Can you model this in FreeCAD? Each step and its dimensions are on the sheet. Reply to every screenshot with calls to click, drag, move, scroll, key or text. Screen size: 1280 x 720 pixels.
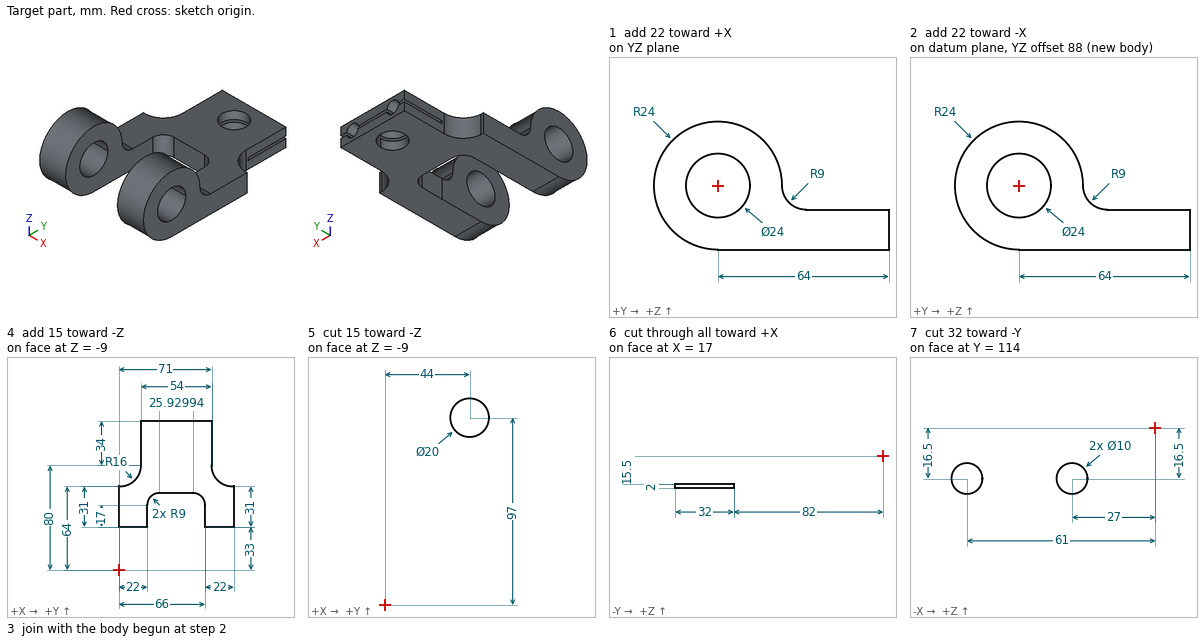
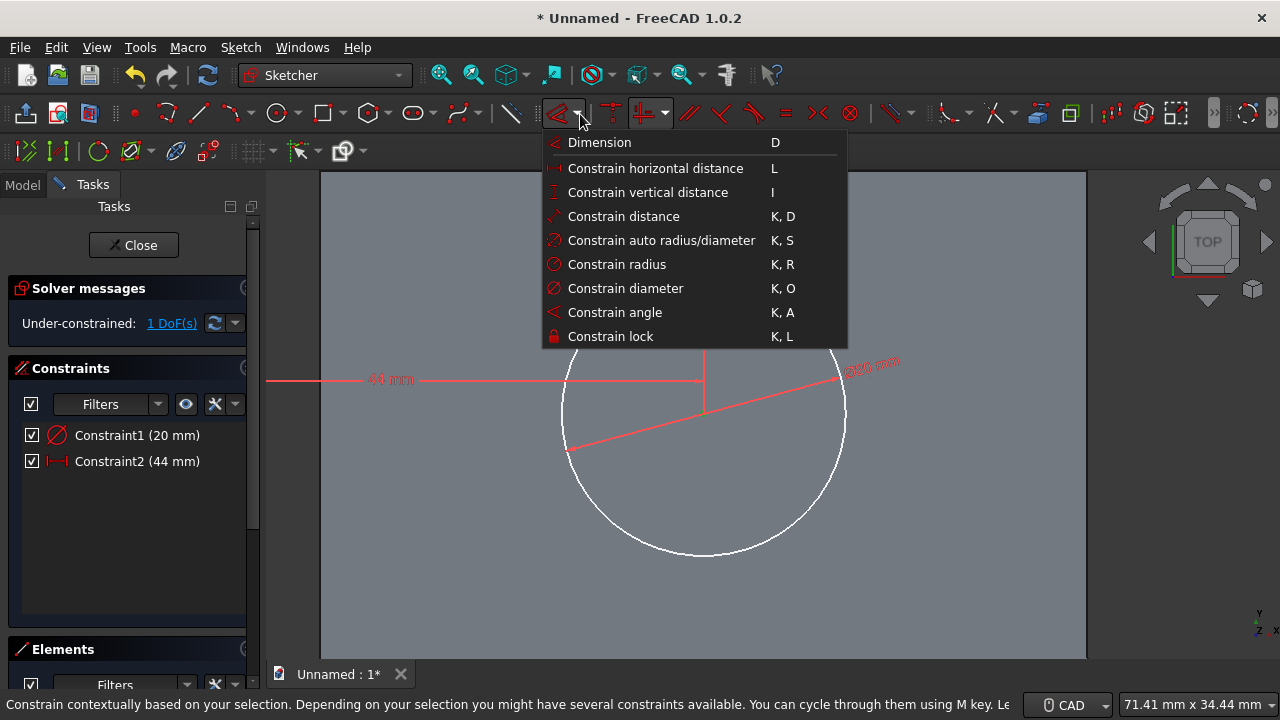
click(695, 192)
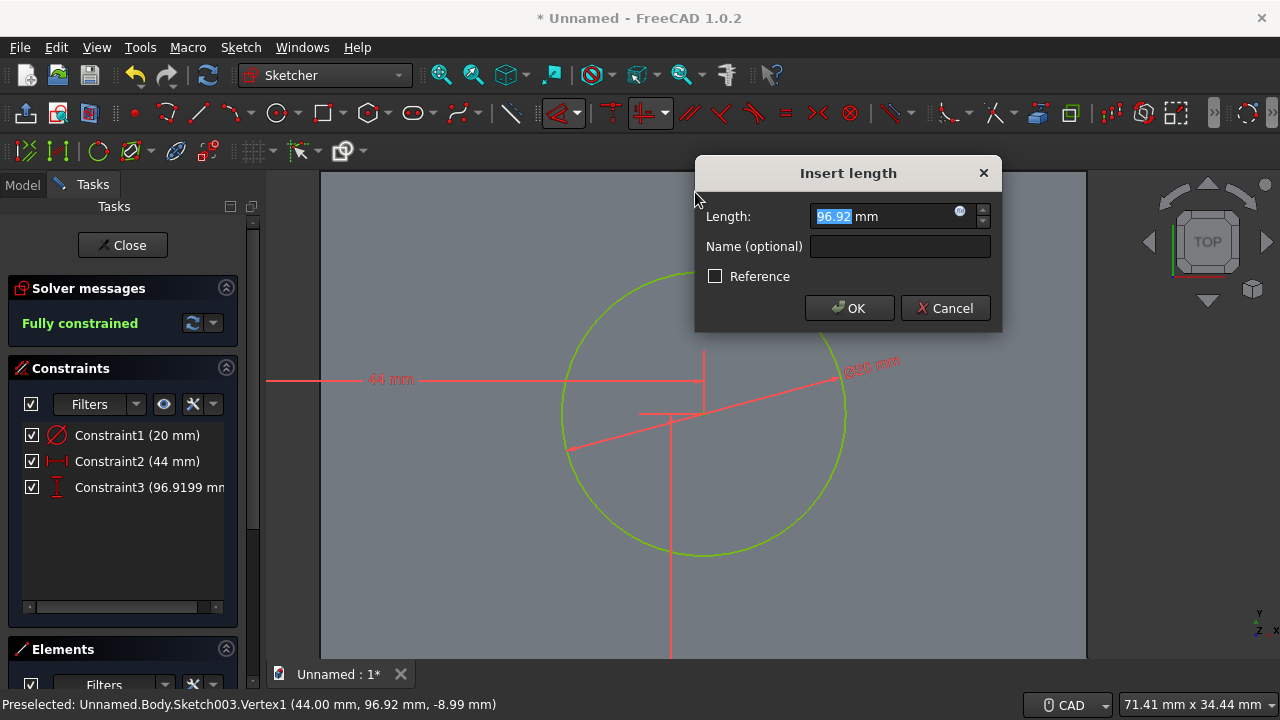
text(97)
key(Return)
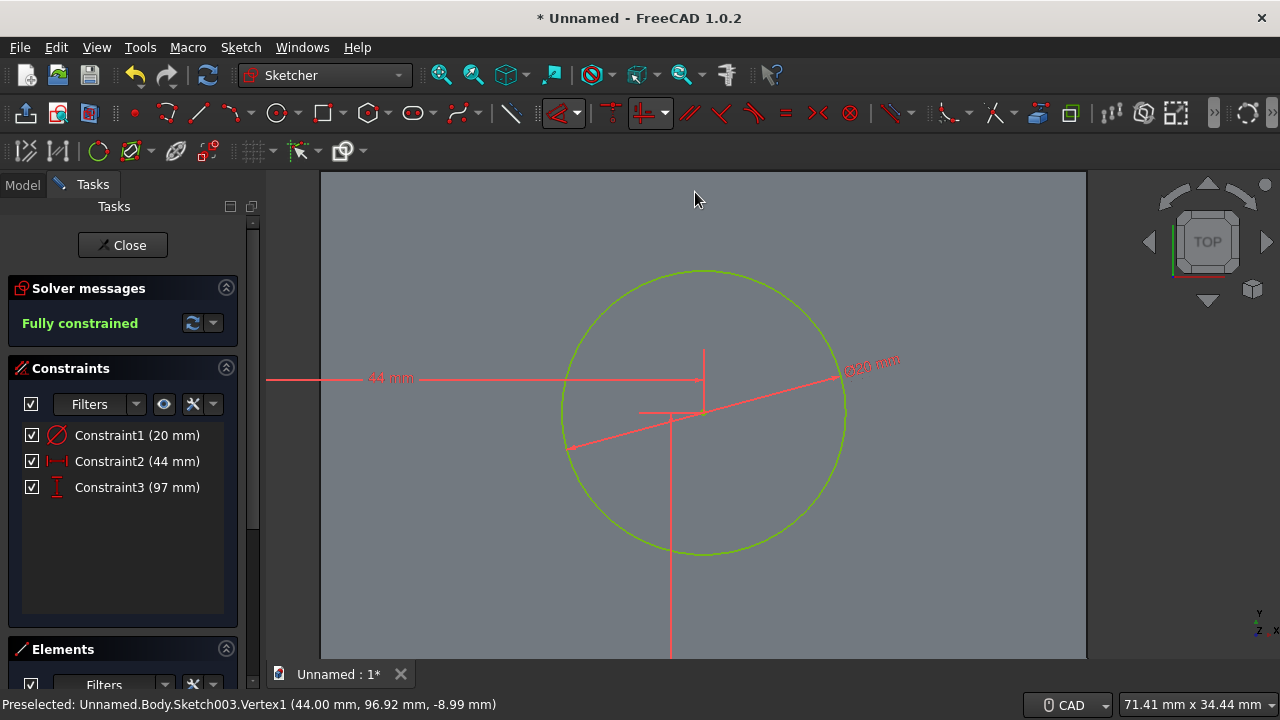
click(123, 245)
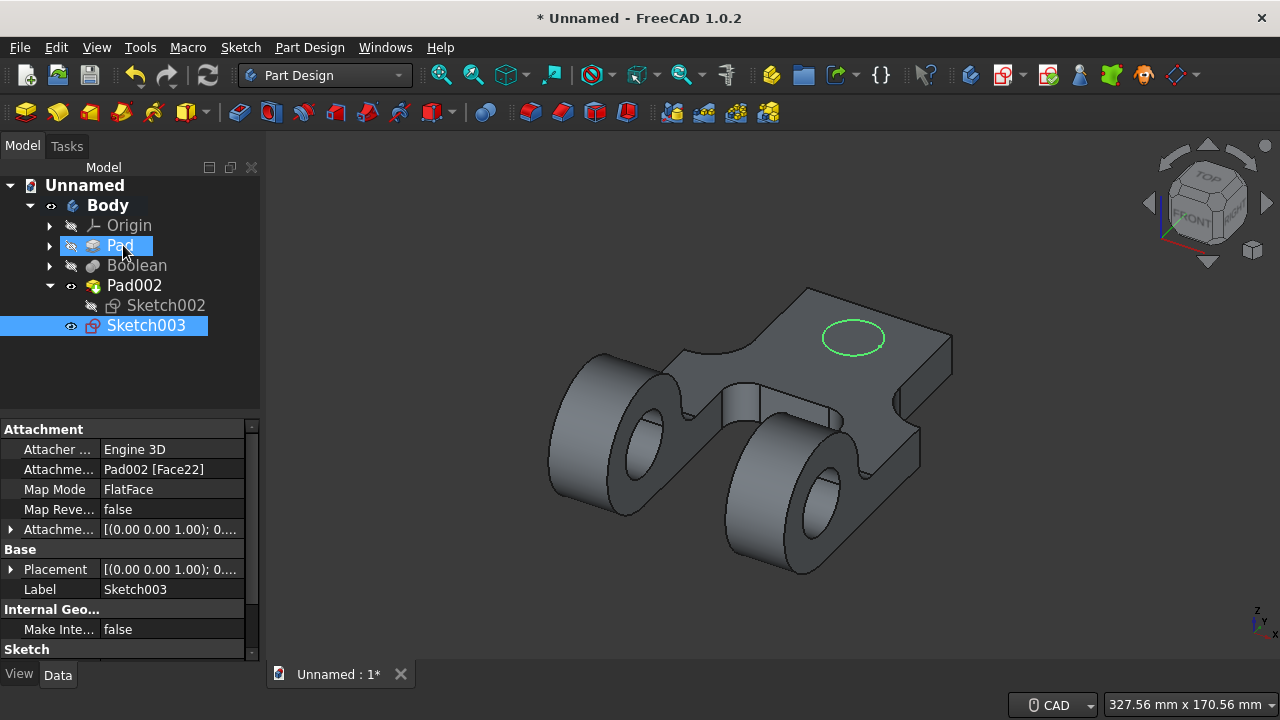
click(240, 112)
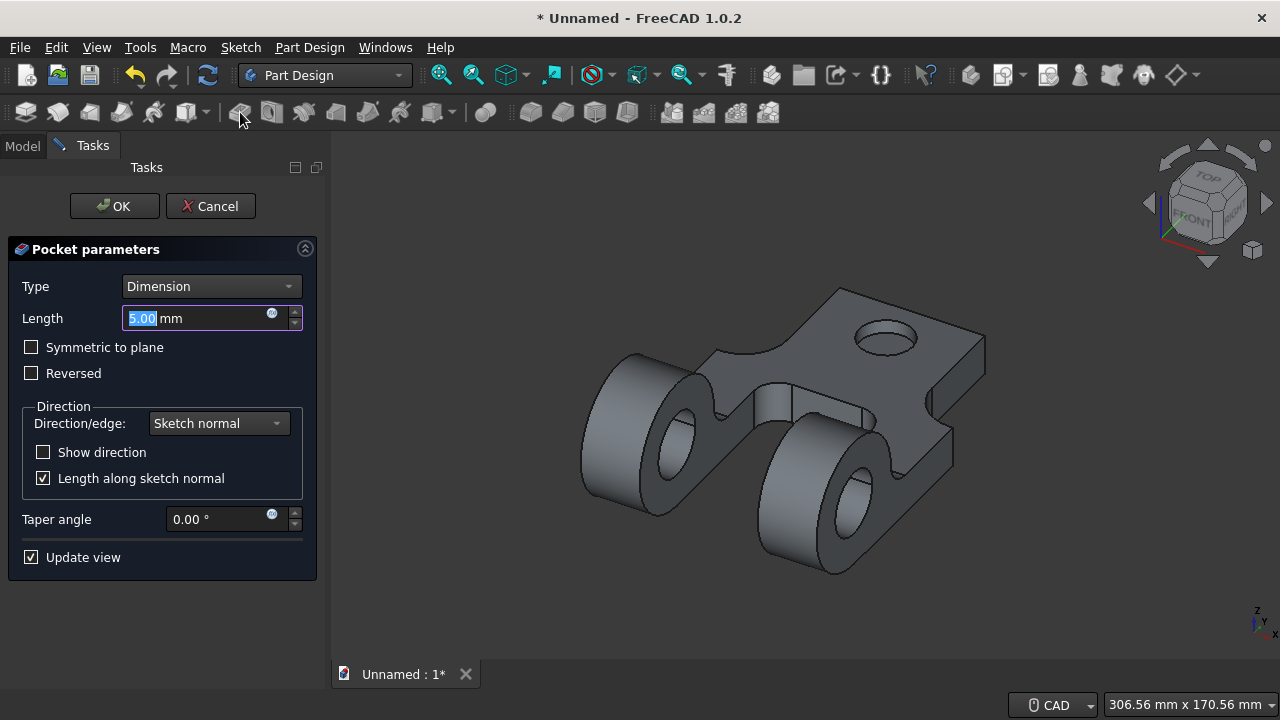
text(15)
key(Tab)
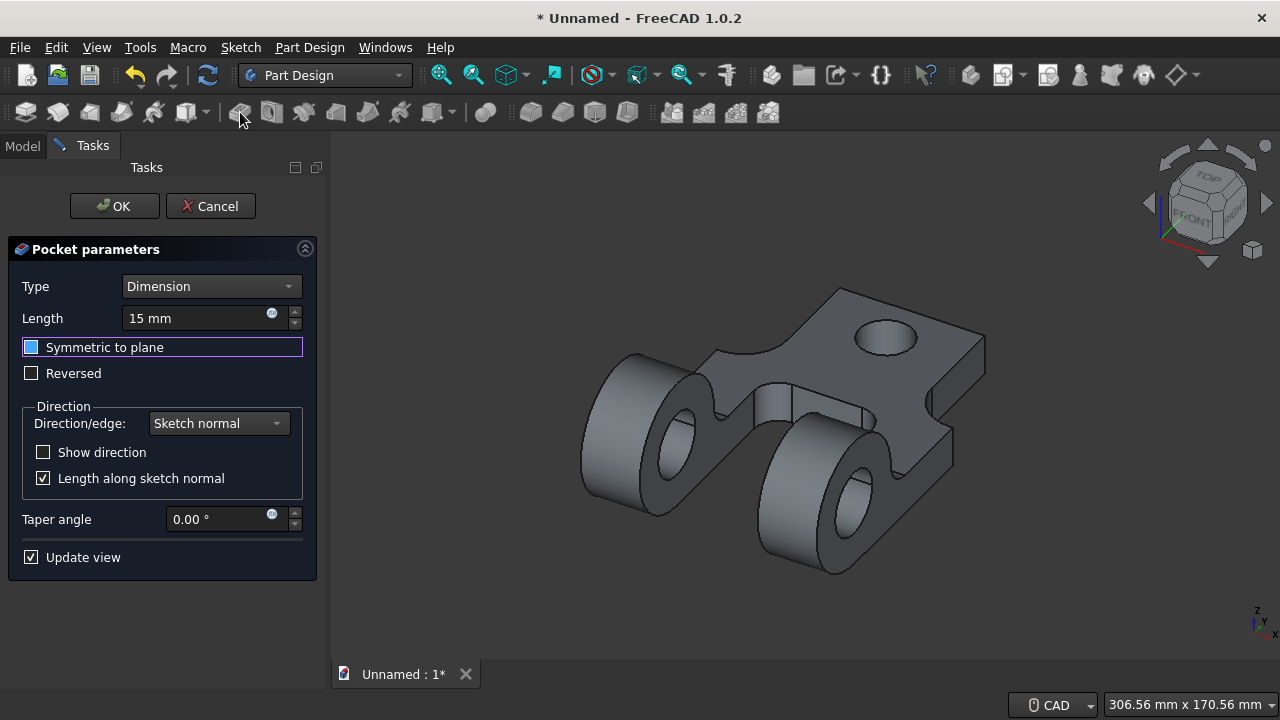
click(115, 206)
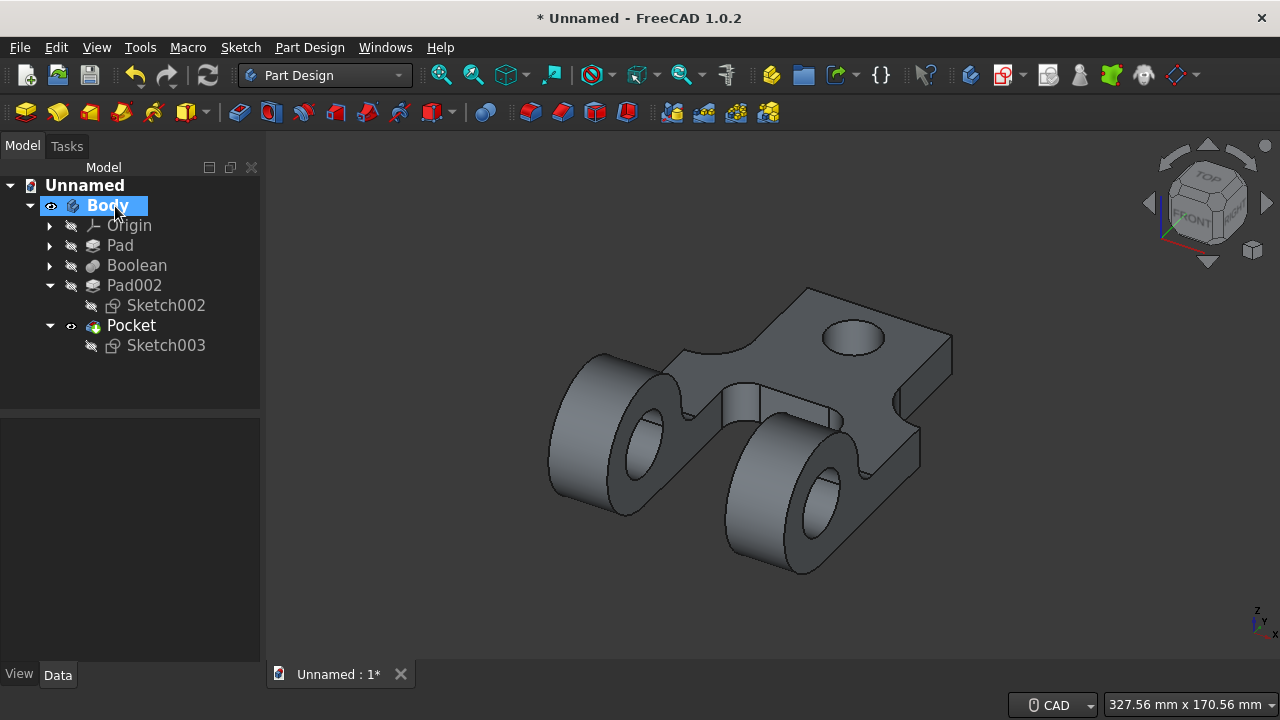
key(6)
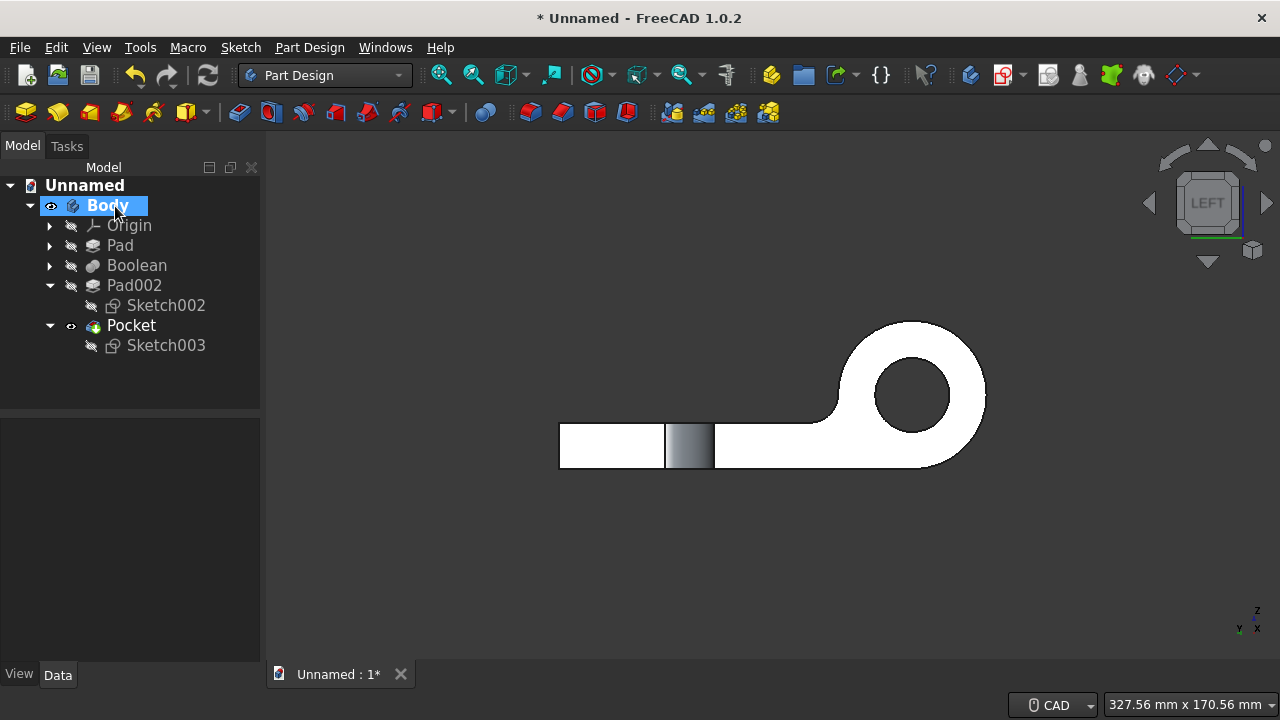
click(442, 76)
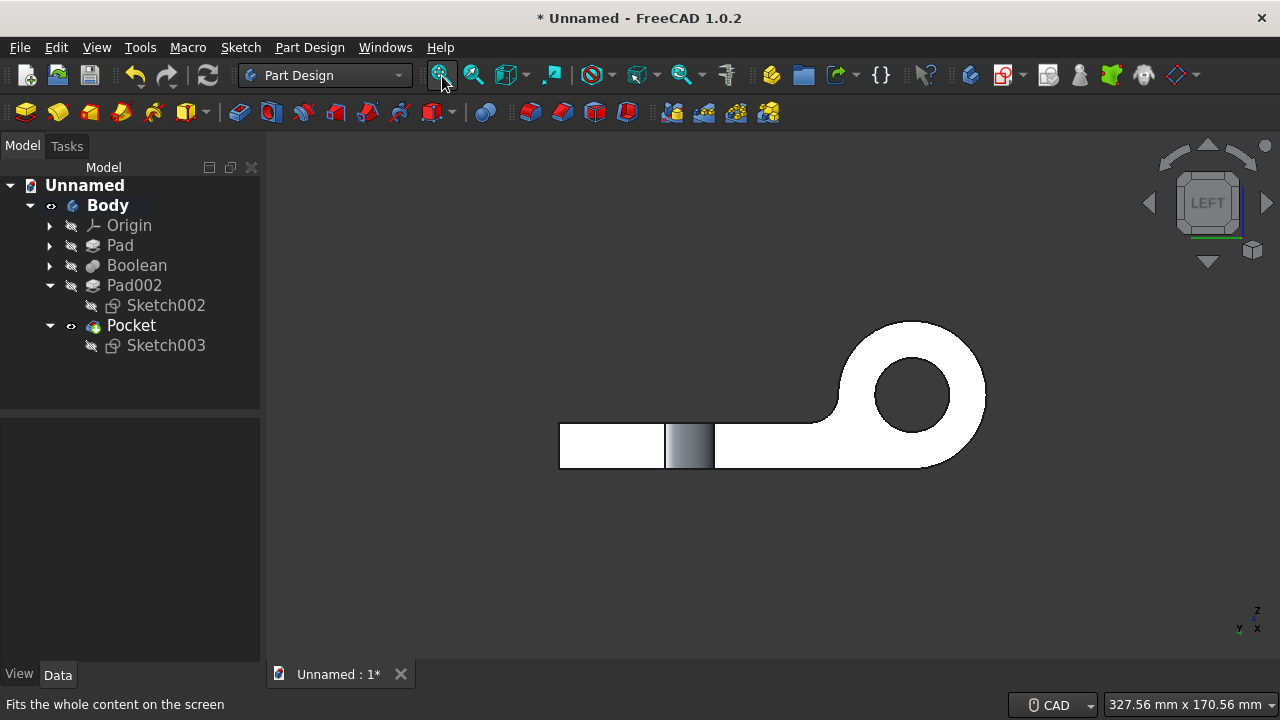
click(597, 445)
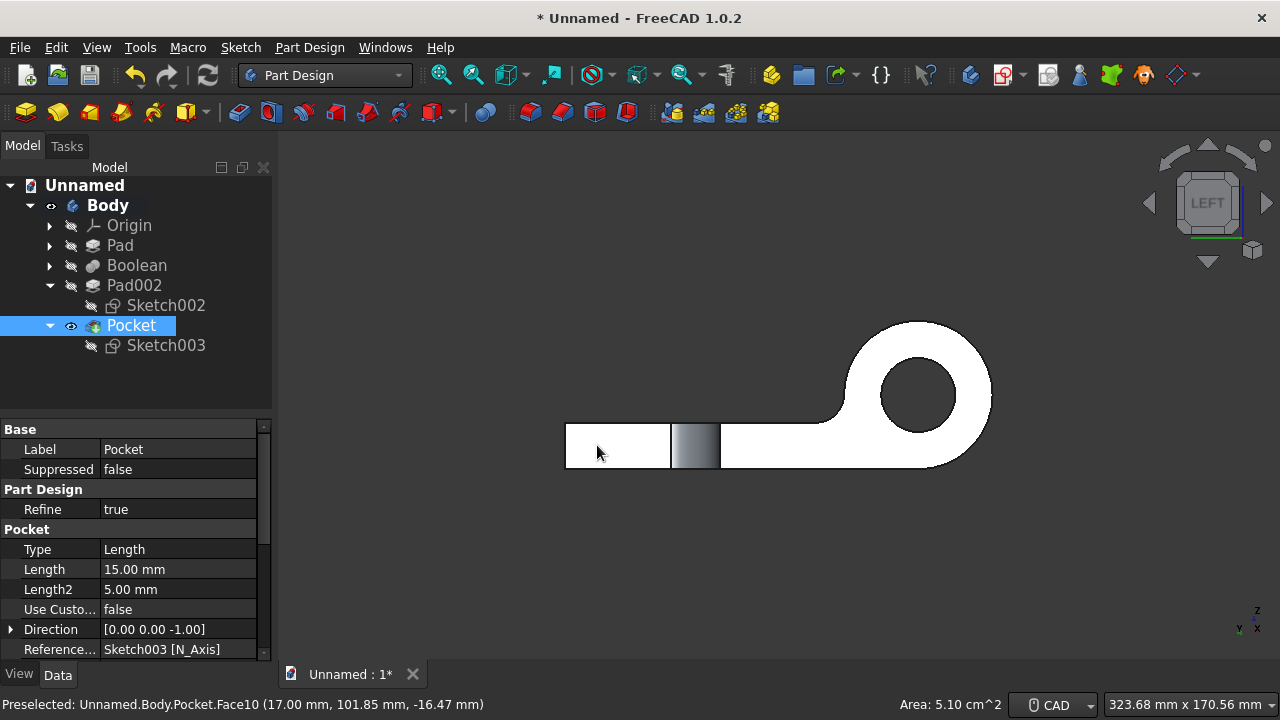
click(1004, 76)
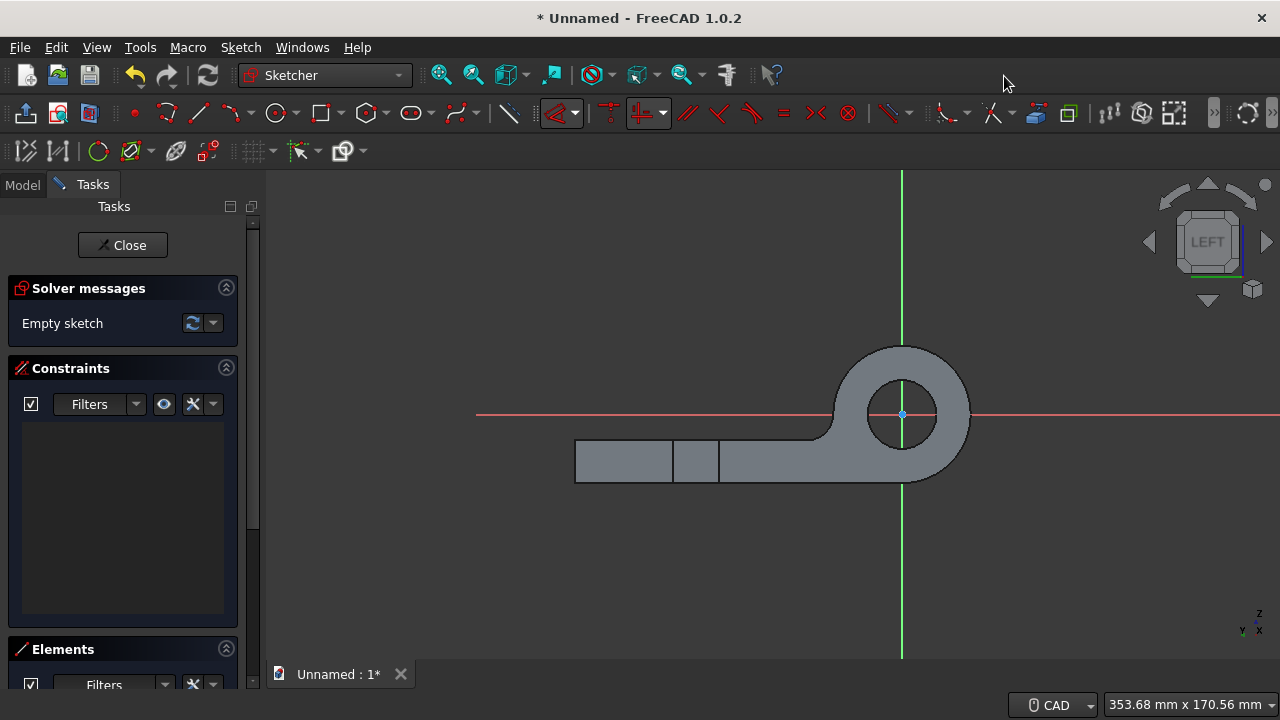
scroll(605, 471, up, 9)